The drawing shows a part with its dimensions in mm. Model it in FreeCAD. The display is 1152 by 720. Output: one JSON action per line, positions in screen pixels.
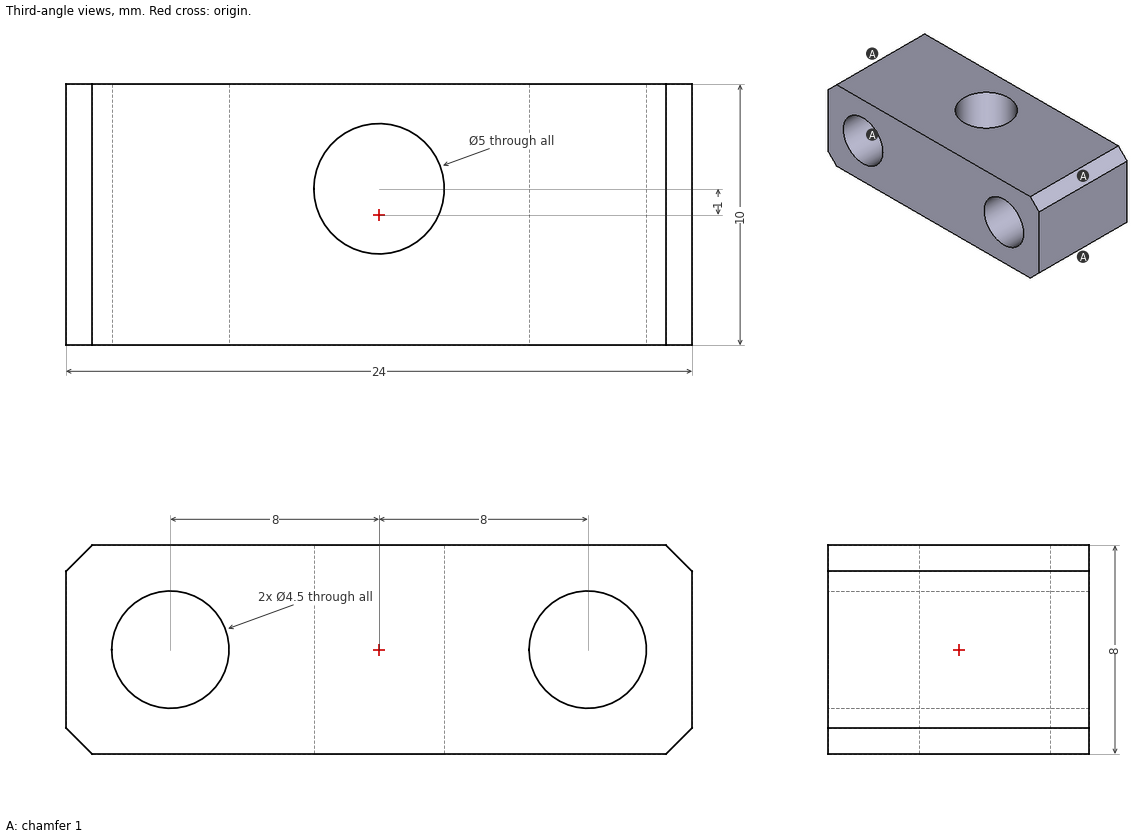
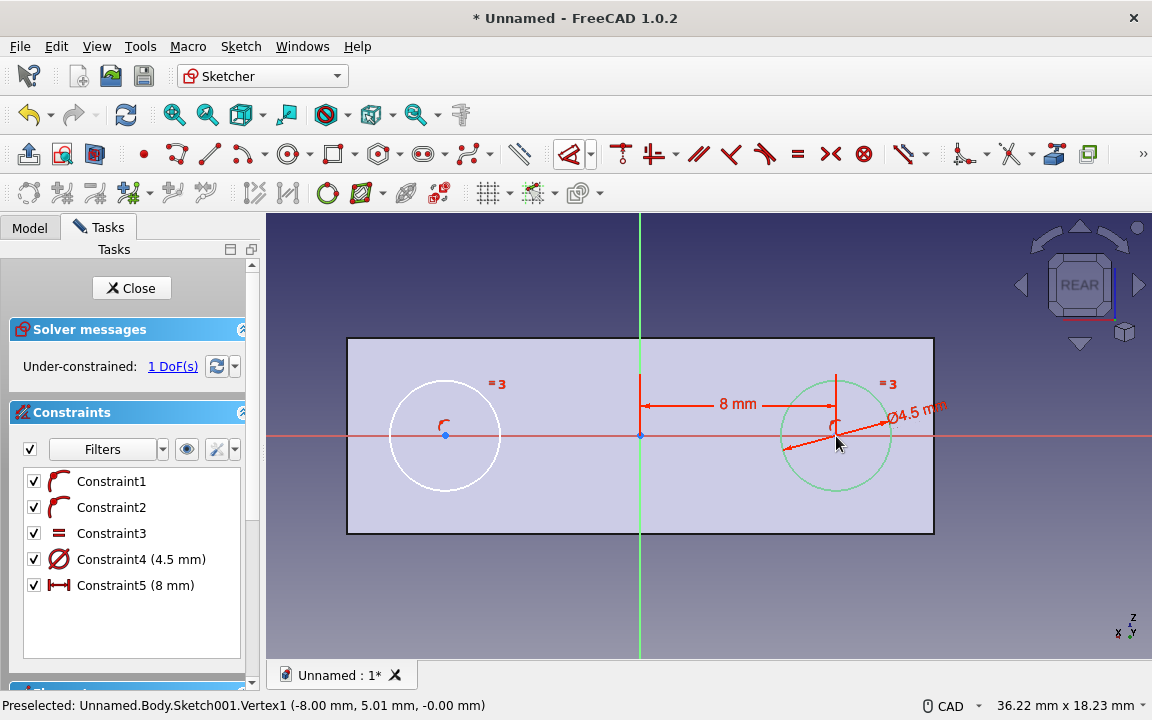
{"action": "left_click", "coordinate": [445, 436]}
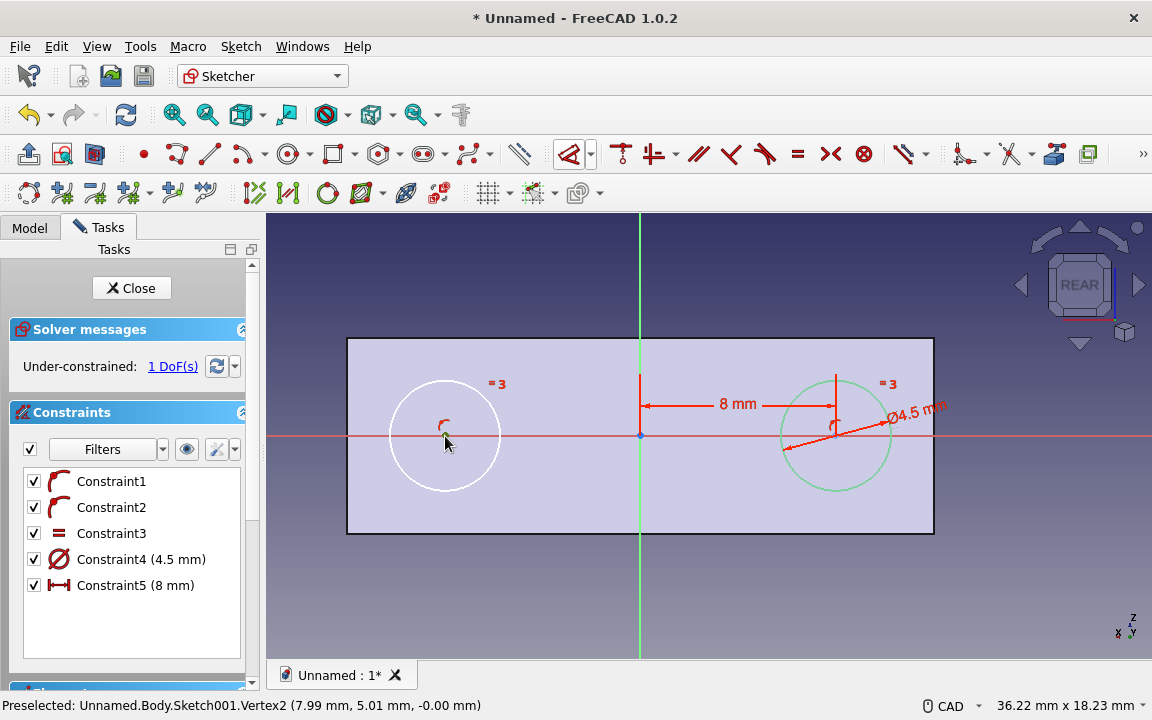
{"action": "key", "text": "l"}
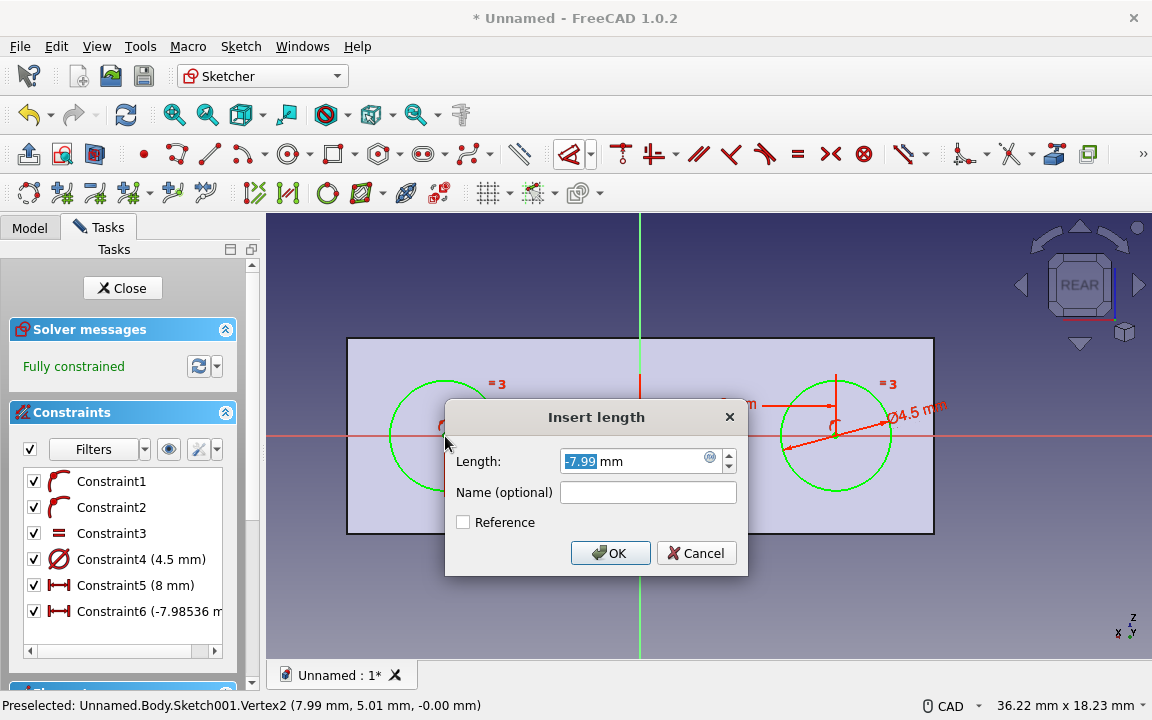
{"action": "type", "text": "-8"}
{"action": "key", "text": "Return"}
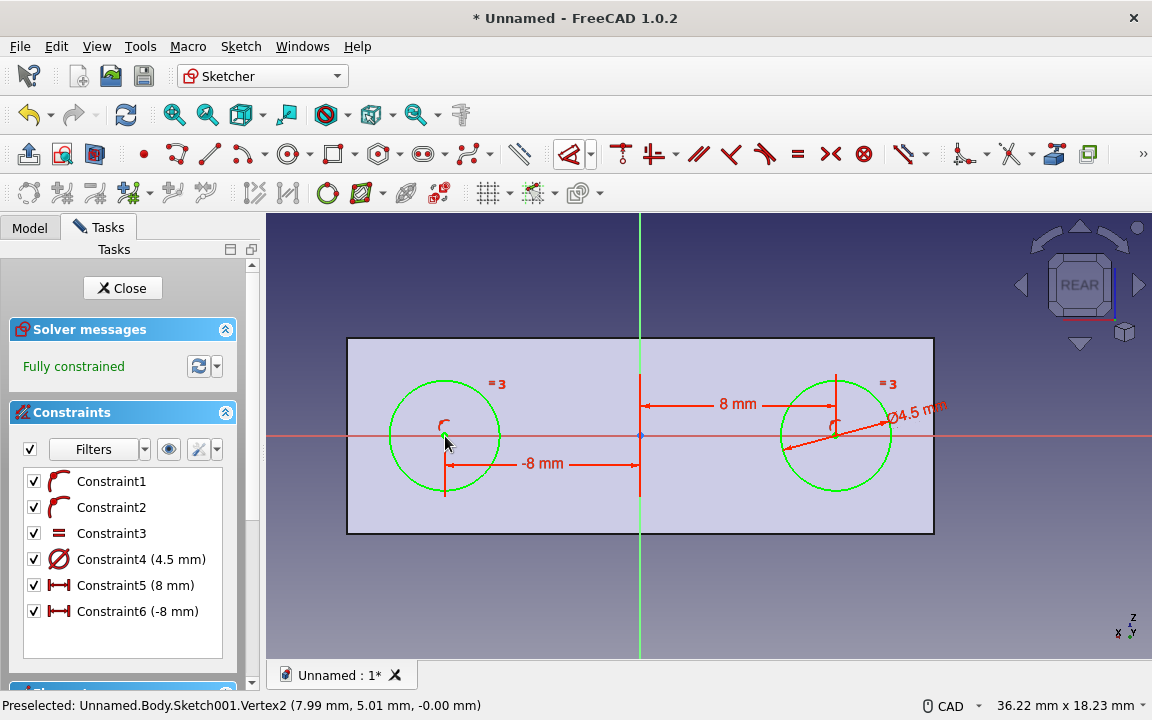
{"action": "left_click", "coordinate": [123, 288]}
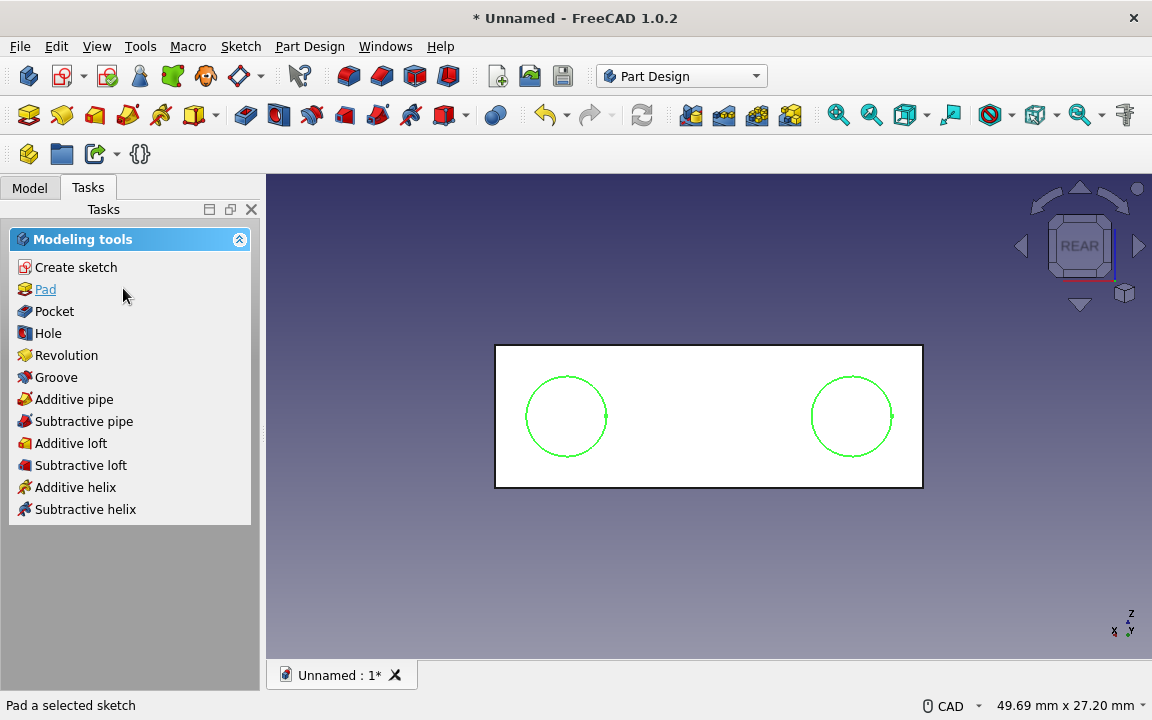
{"action": "left_click", "coordinate": [279, 116]}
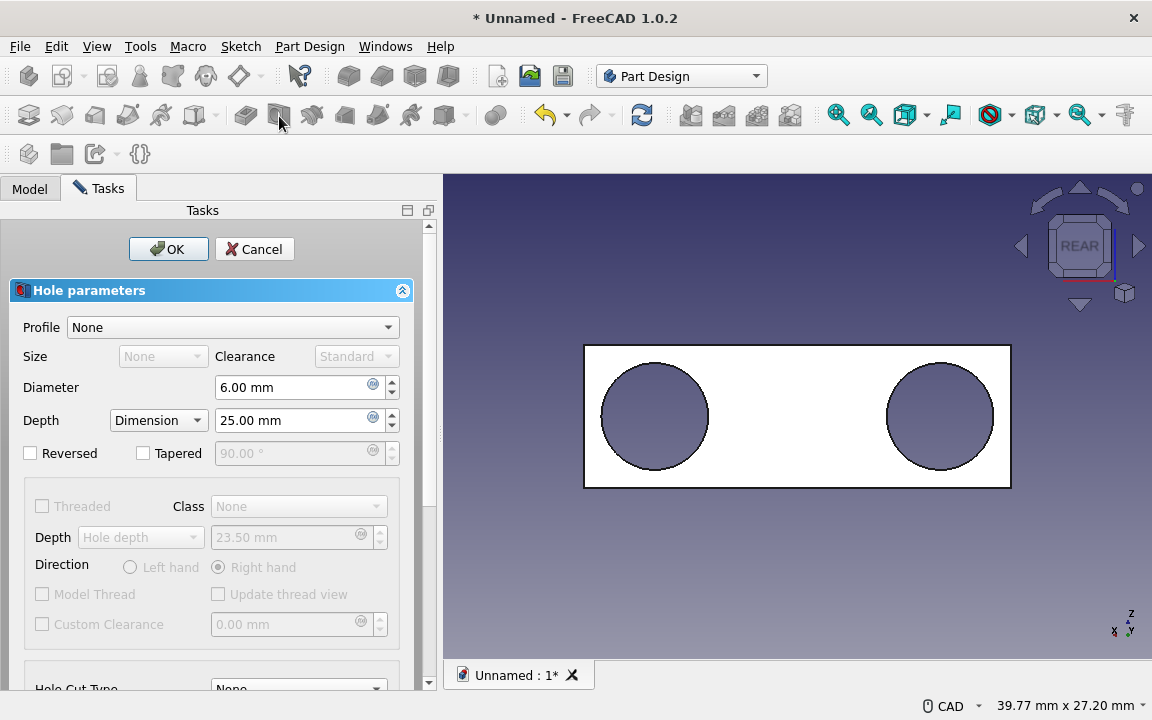
{"action": "triple_click", "coordinate": [300, 388]}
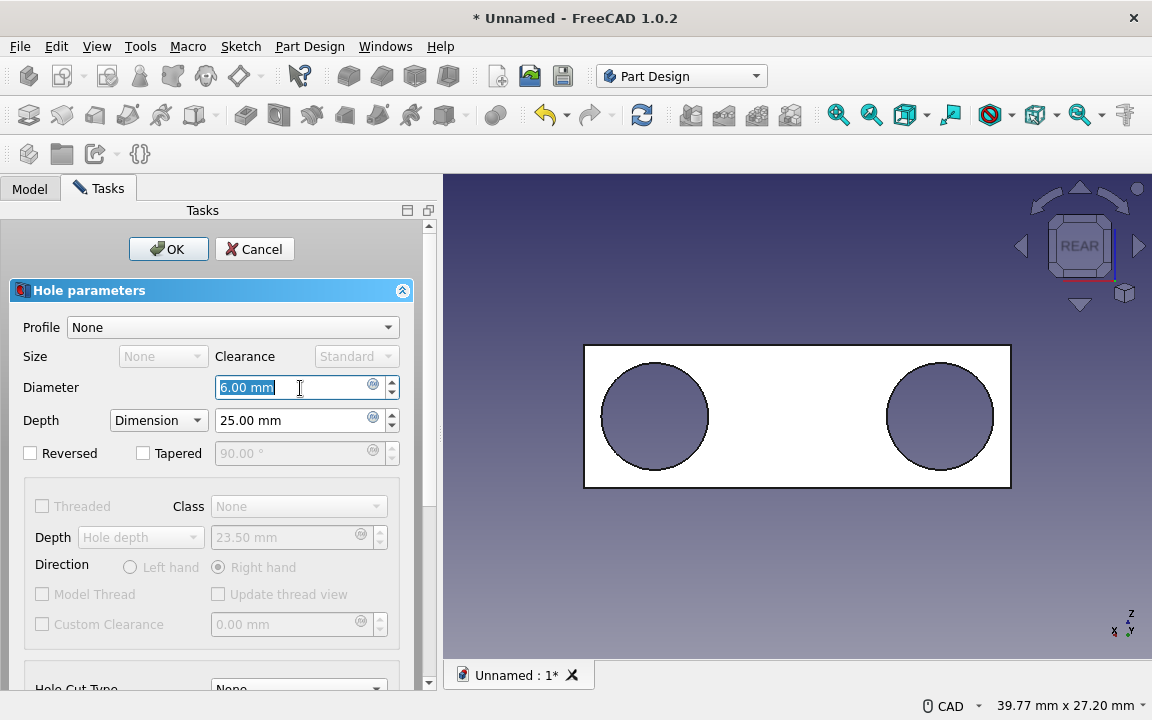
{"action": "type", "text": "4.5"}
{"action": "key", "text": "Tab"}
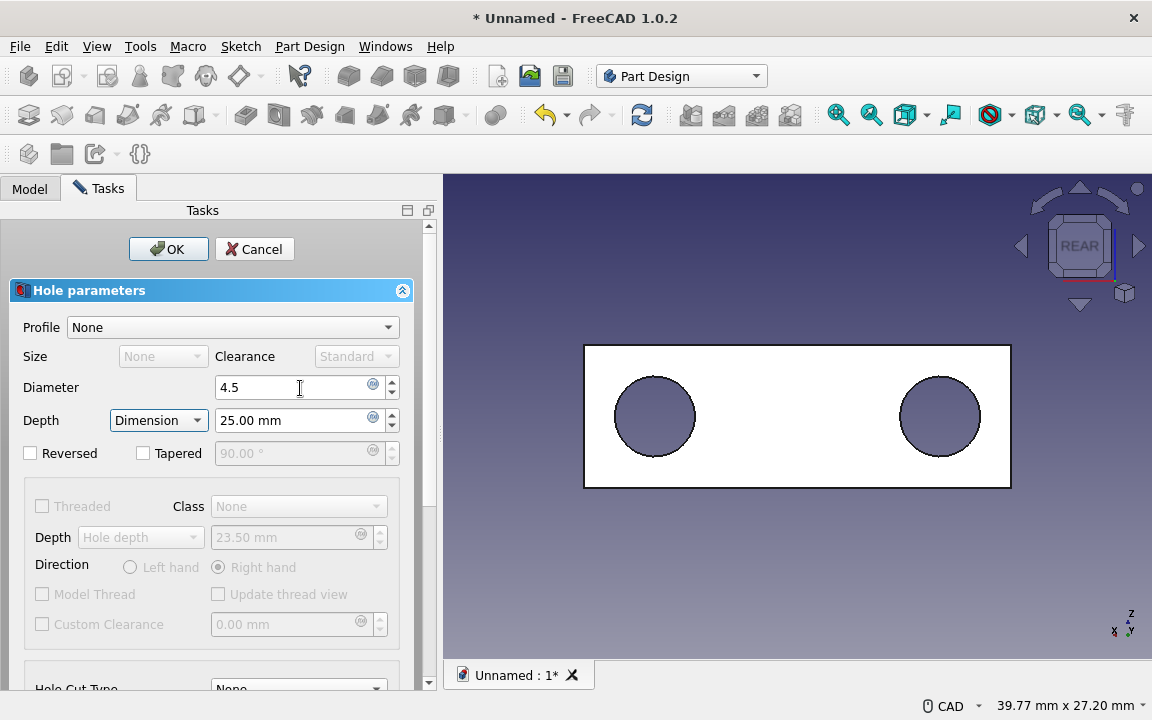
{"action": "left_click", "coordinate": [160, 420]}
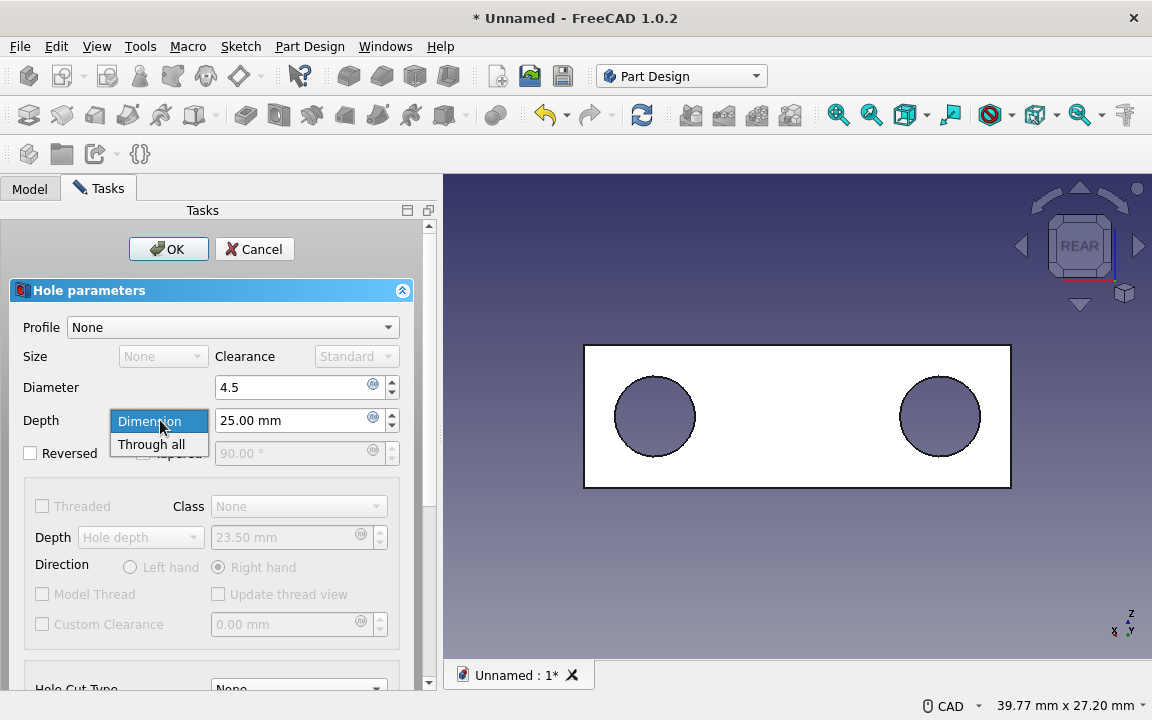
{"action": "left_click", "coordinate": [158, 444]}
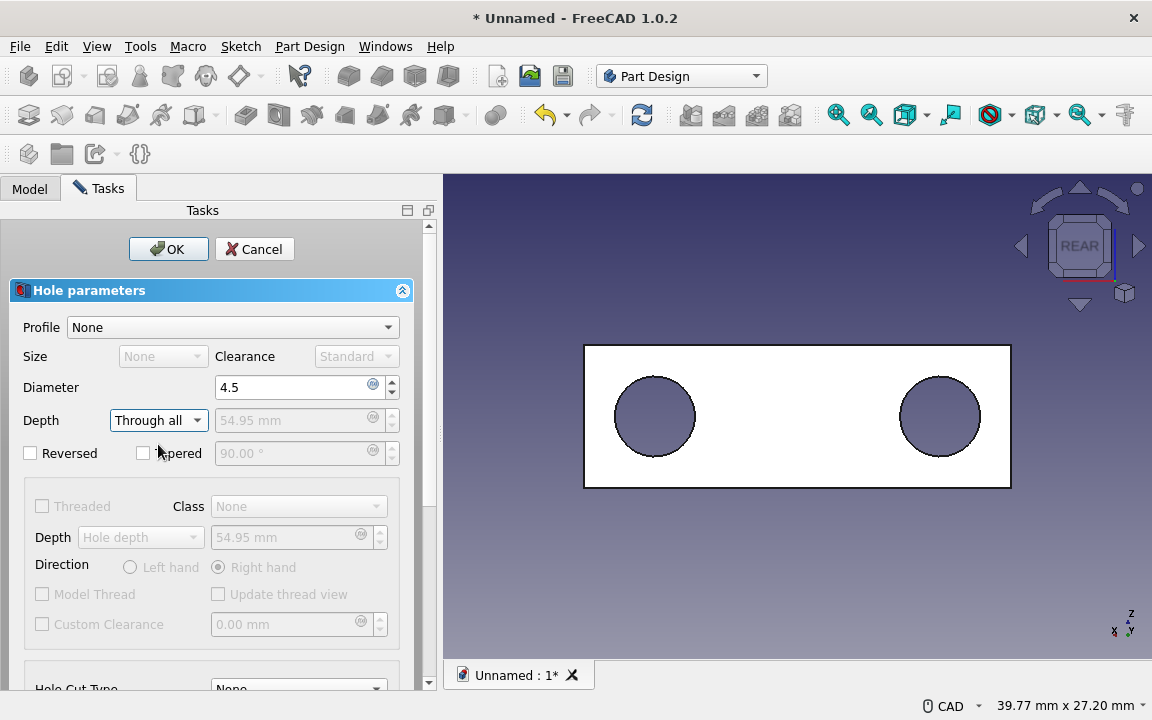
{"action": "left_click", "coordinate": [169, 249]}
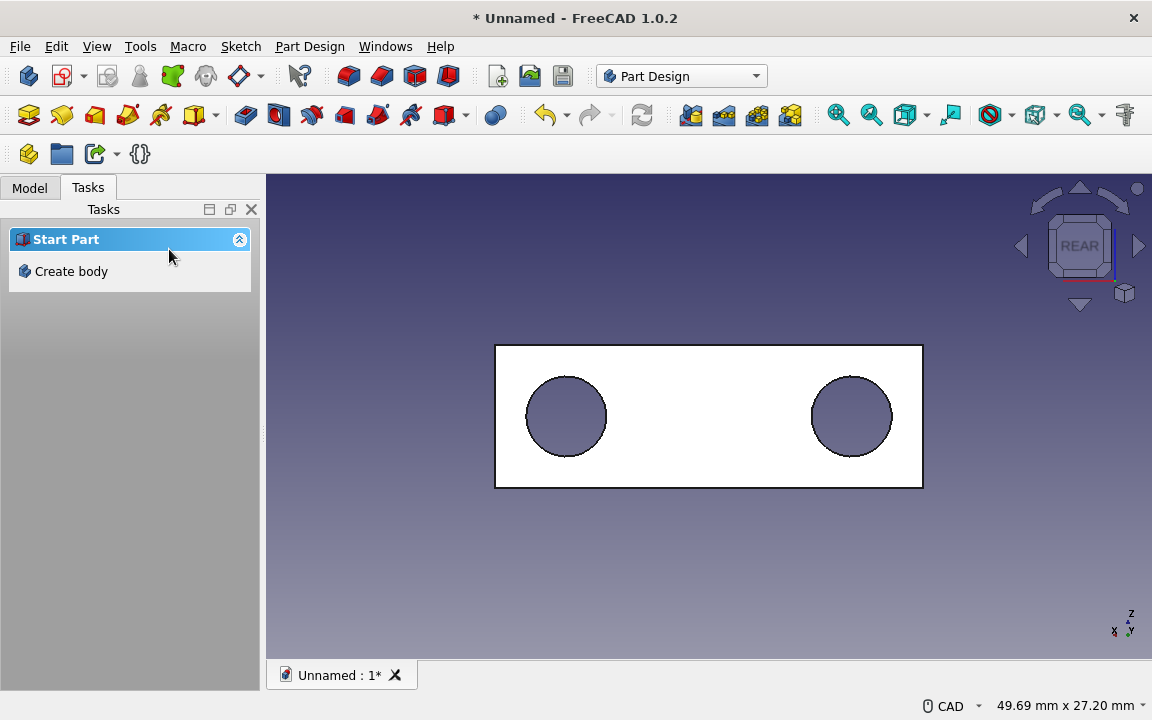
{"action": "key", "text": "0"}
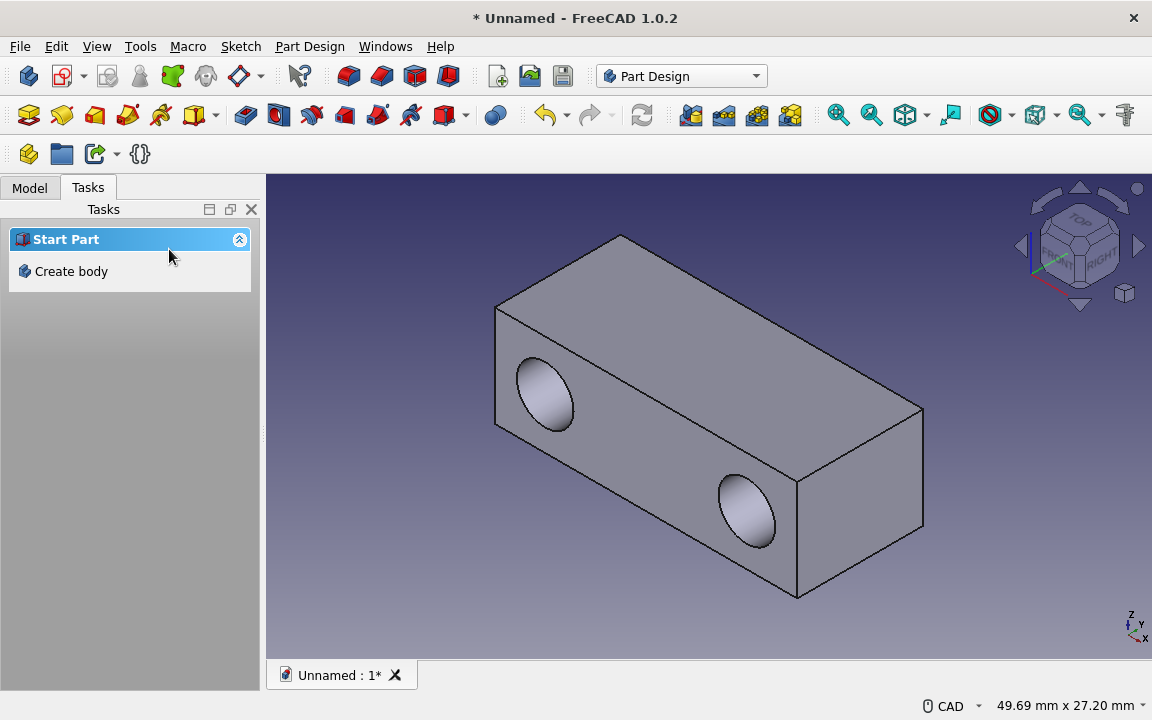
{"action": "left_click", "coordinate": [860, 445]}